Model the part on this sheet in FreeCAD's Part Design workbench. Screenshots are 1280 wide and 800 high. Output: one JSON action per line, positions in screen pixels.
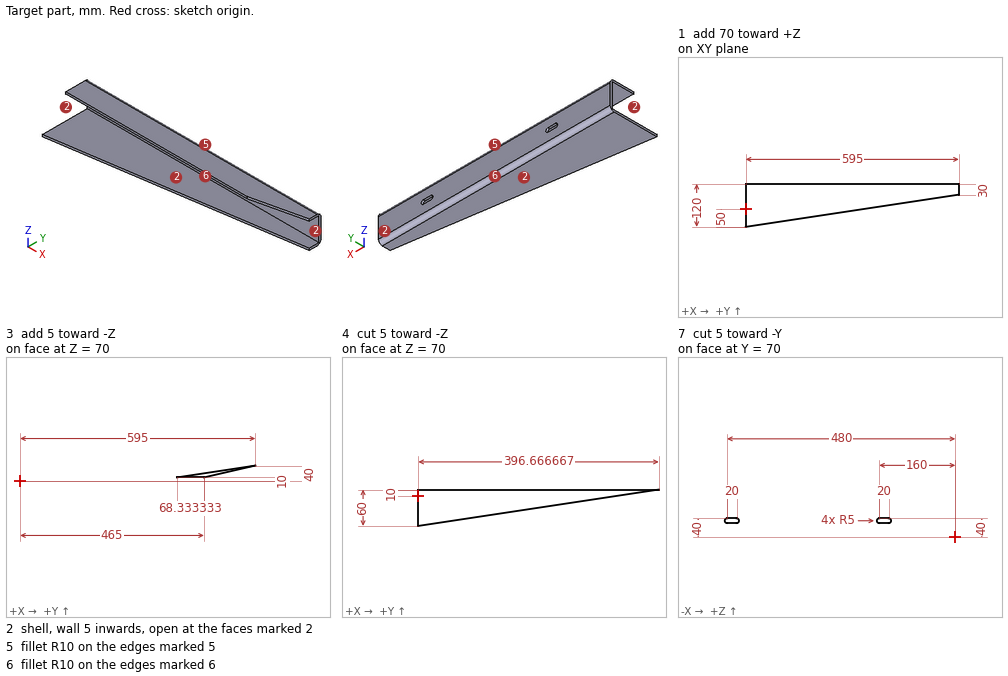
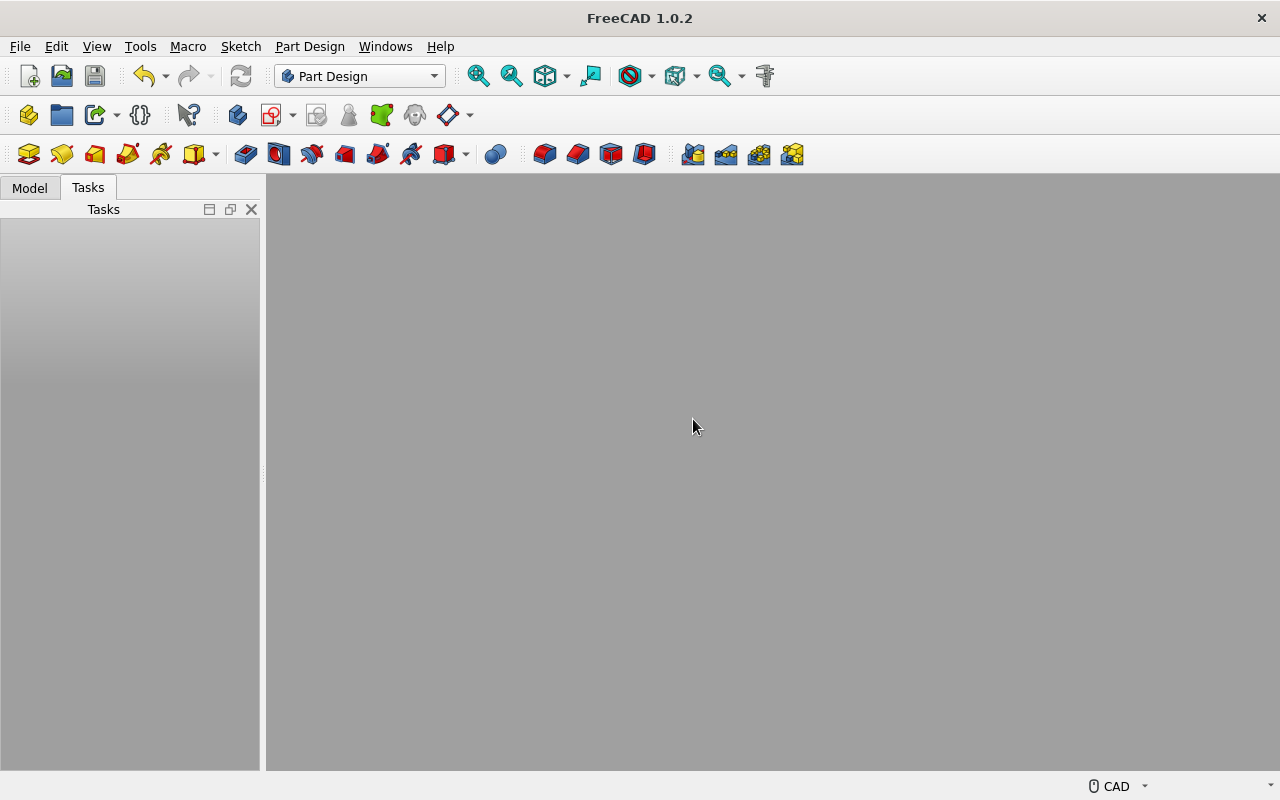
{"action": "key", "text": "ctrl+n"}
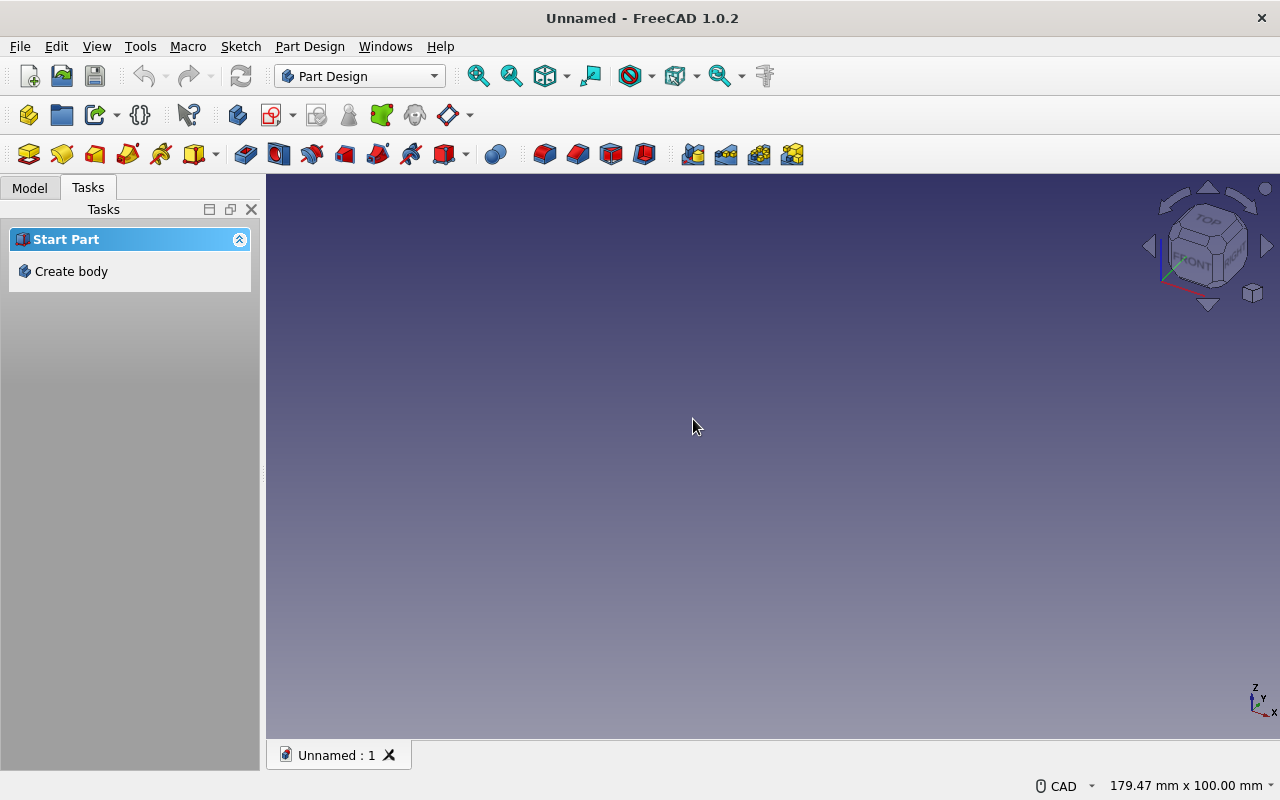
{"action": "left_click", "coordinate": [270, 116]}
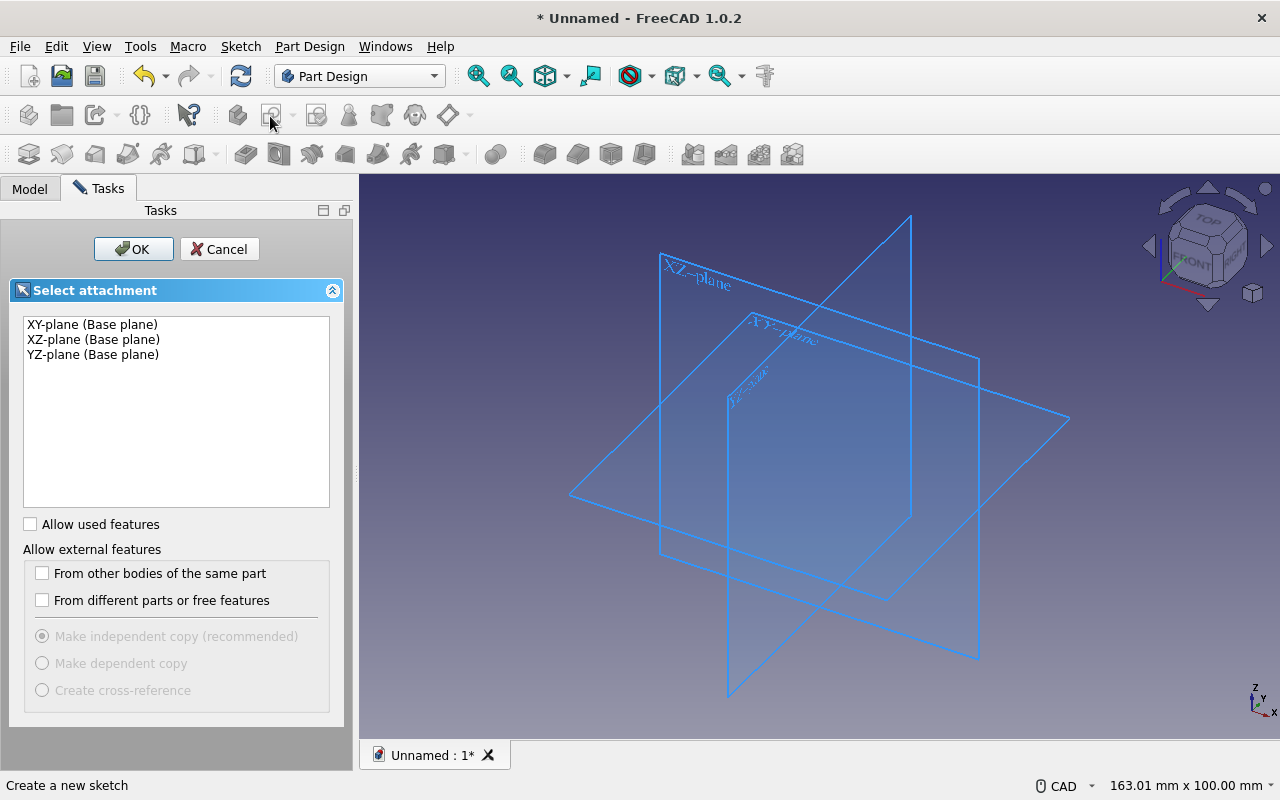
{"action": "left_click", "coordinate": [84, 324]}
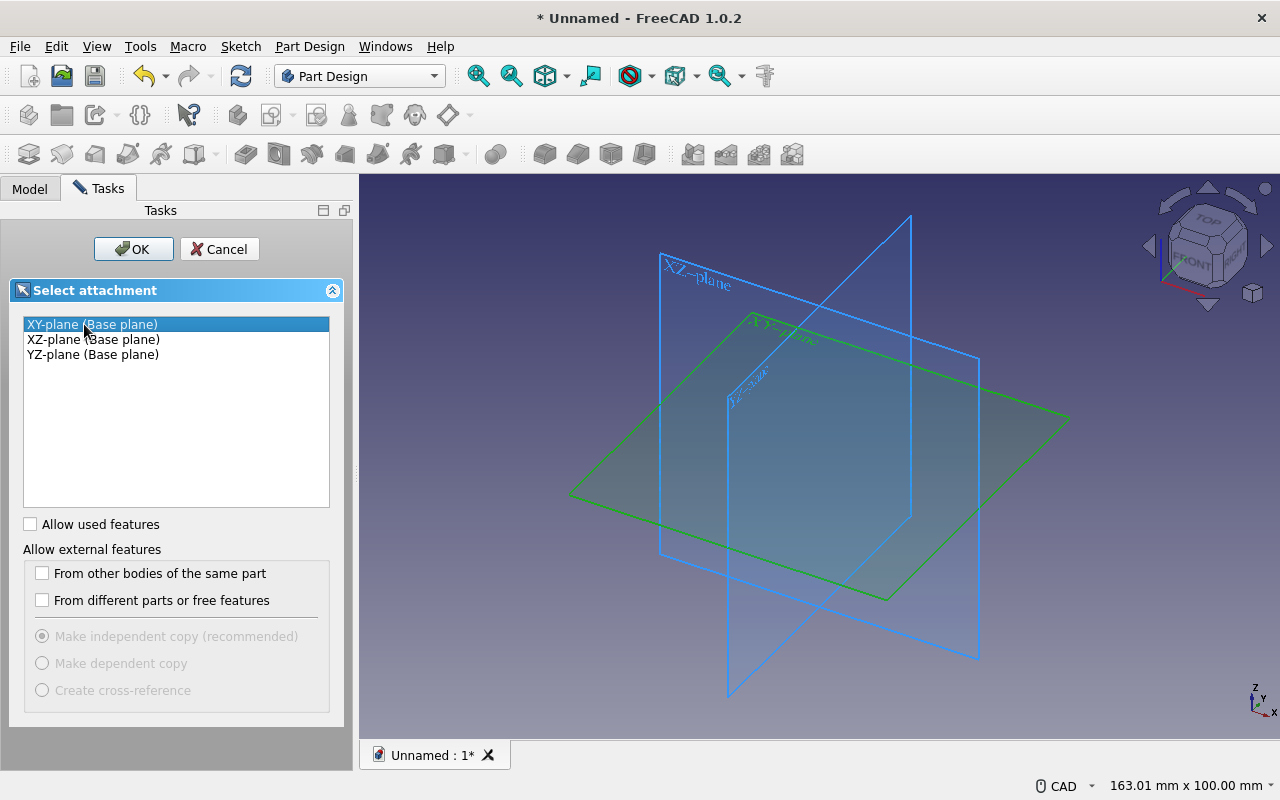
{"action": "left_click", "coordinate": [134, 249]}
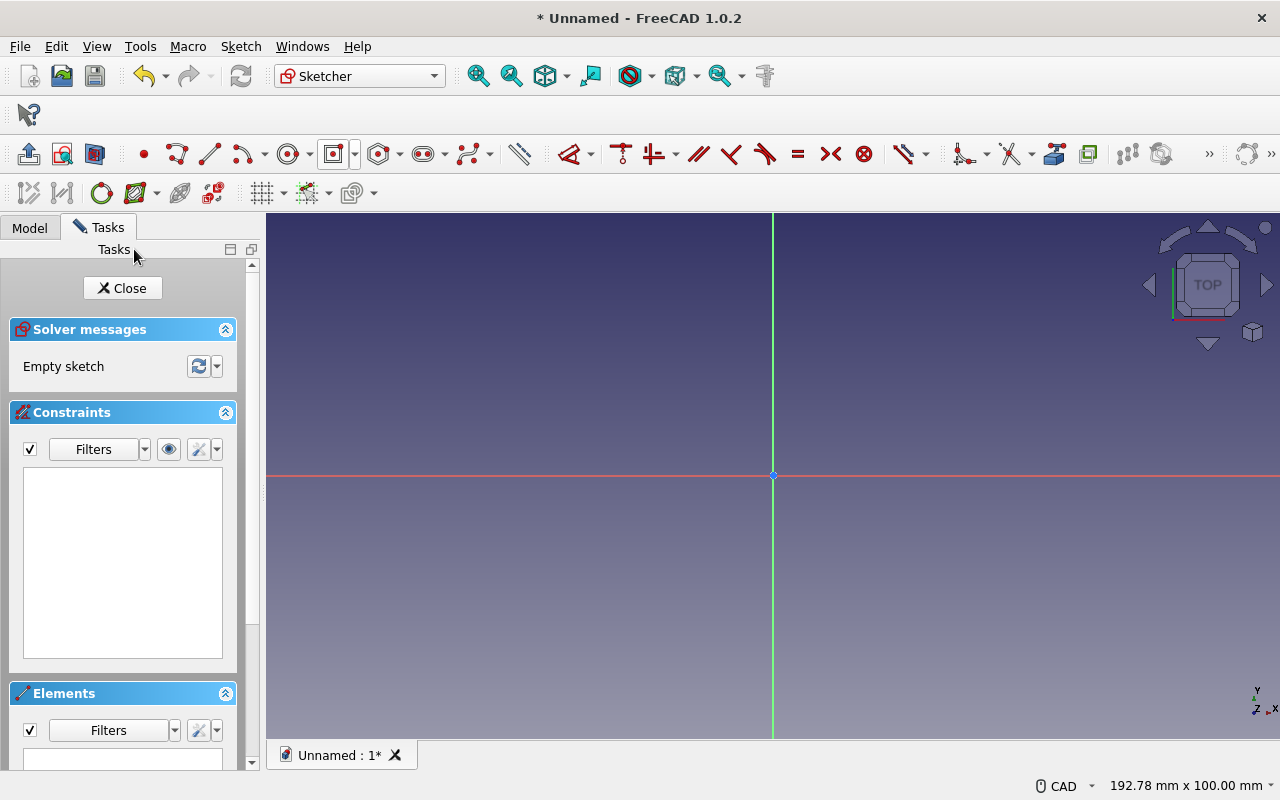
{"action": "scroll", "coordinate": [294, 489], "scroll_direction": "down", "scroll_amount": 8}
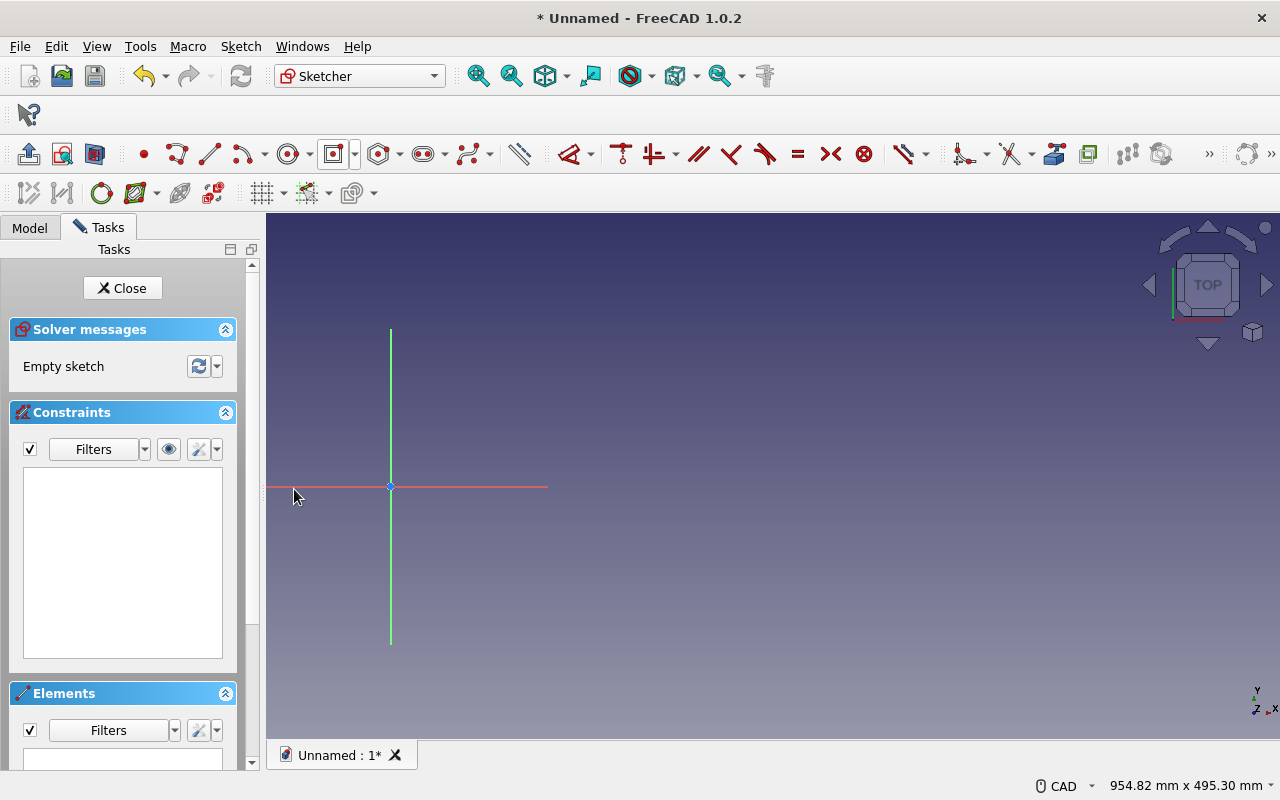
{"action": "key", "text": "g m"}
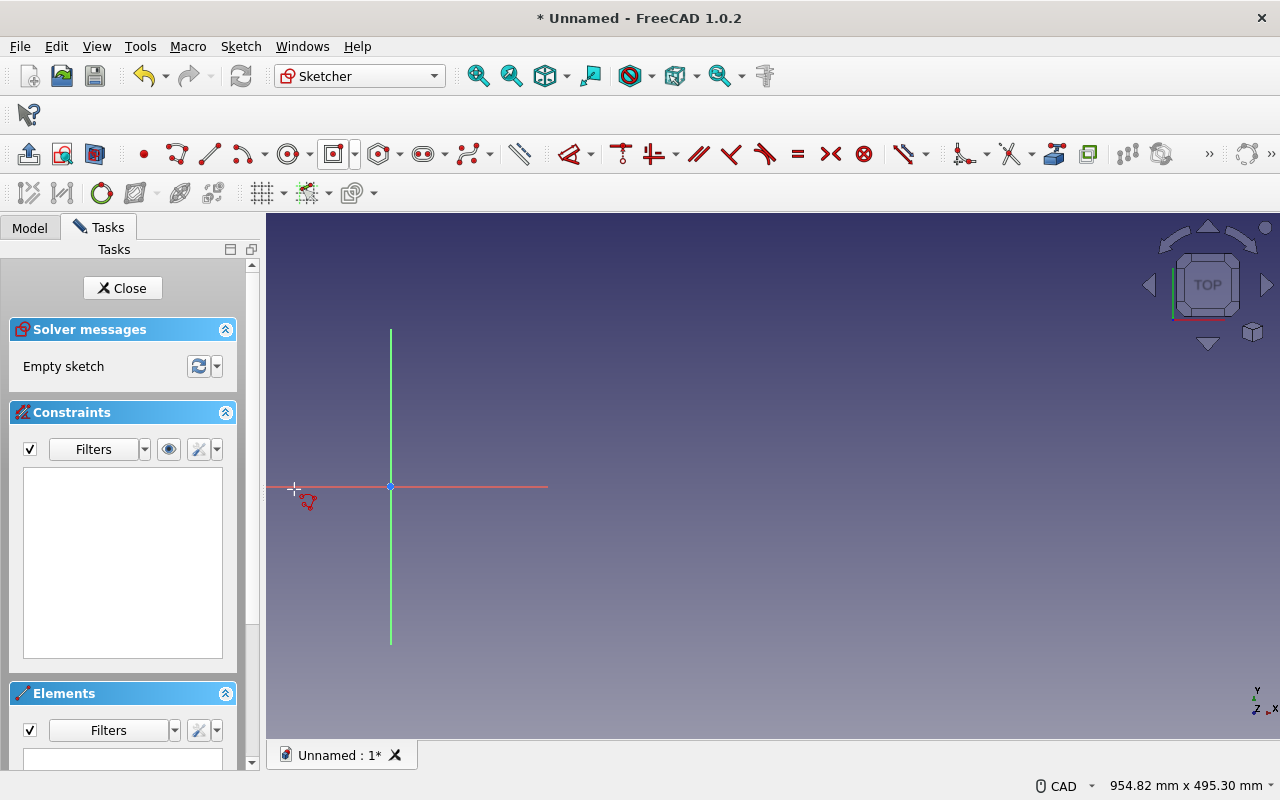
{"action": "left_click", "coordinate": [391, 540]}
{"action": "left_click", "coordinate": [1023, 444]}
{"action": "left_click", "coordinate": [1023, 412]}
{"action": "left_click", "coordinate": [400, 412]}
{"action": "left_click", "coordinate": [391, 541]}
{"action": "key", "text": "Escape"}
{"action": "key", "text": "Escape"}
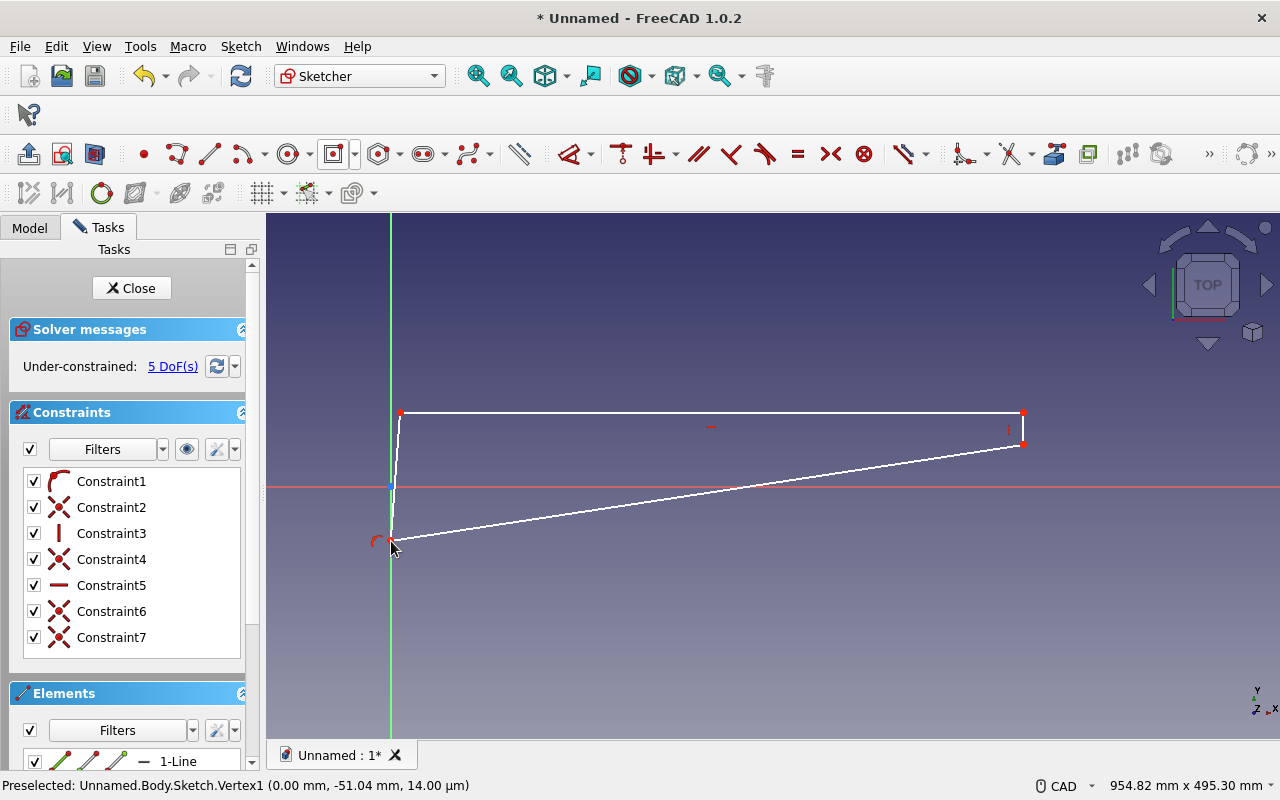
{"action": "left_click", "coordinate": [394, 503]}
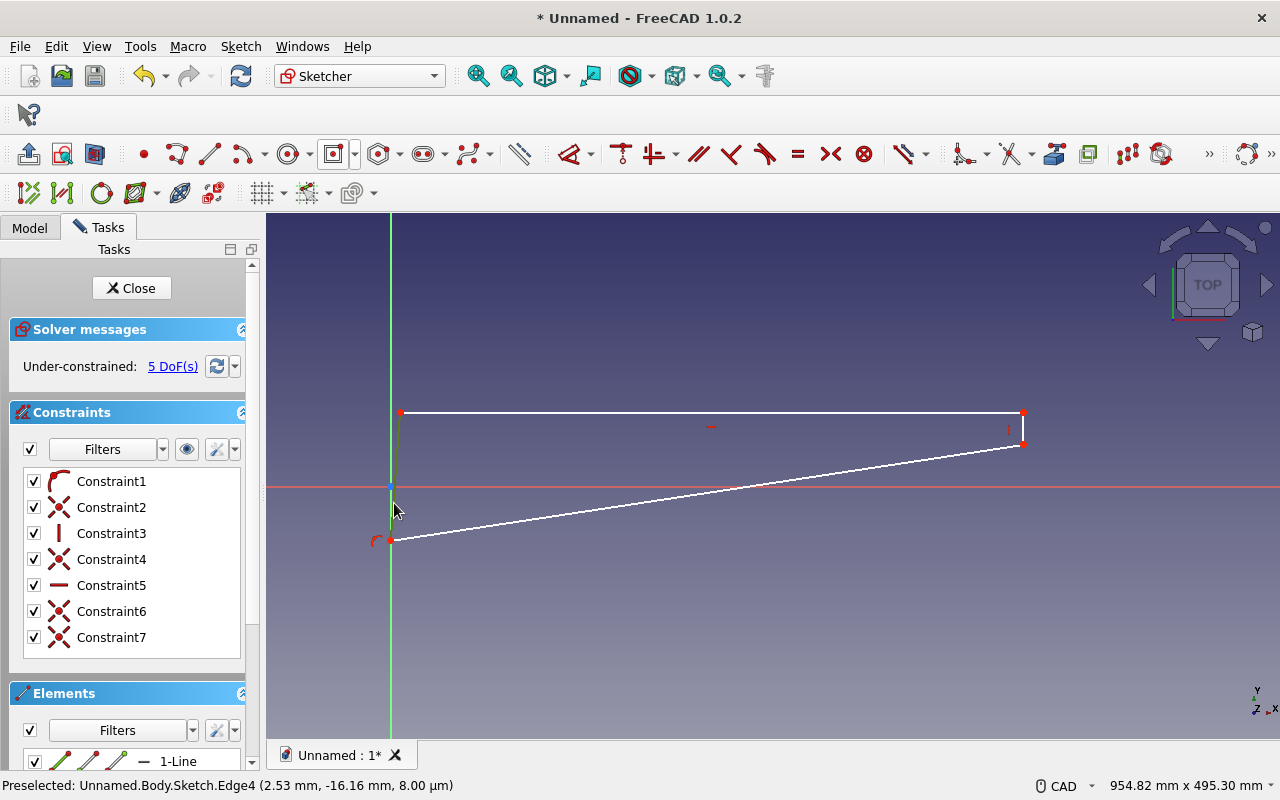
{"action": "key", "text": "v"}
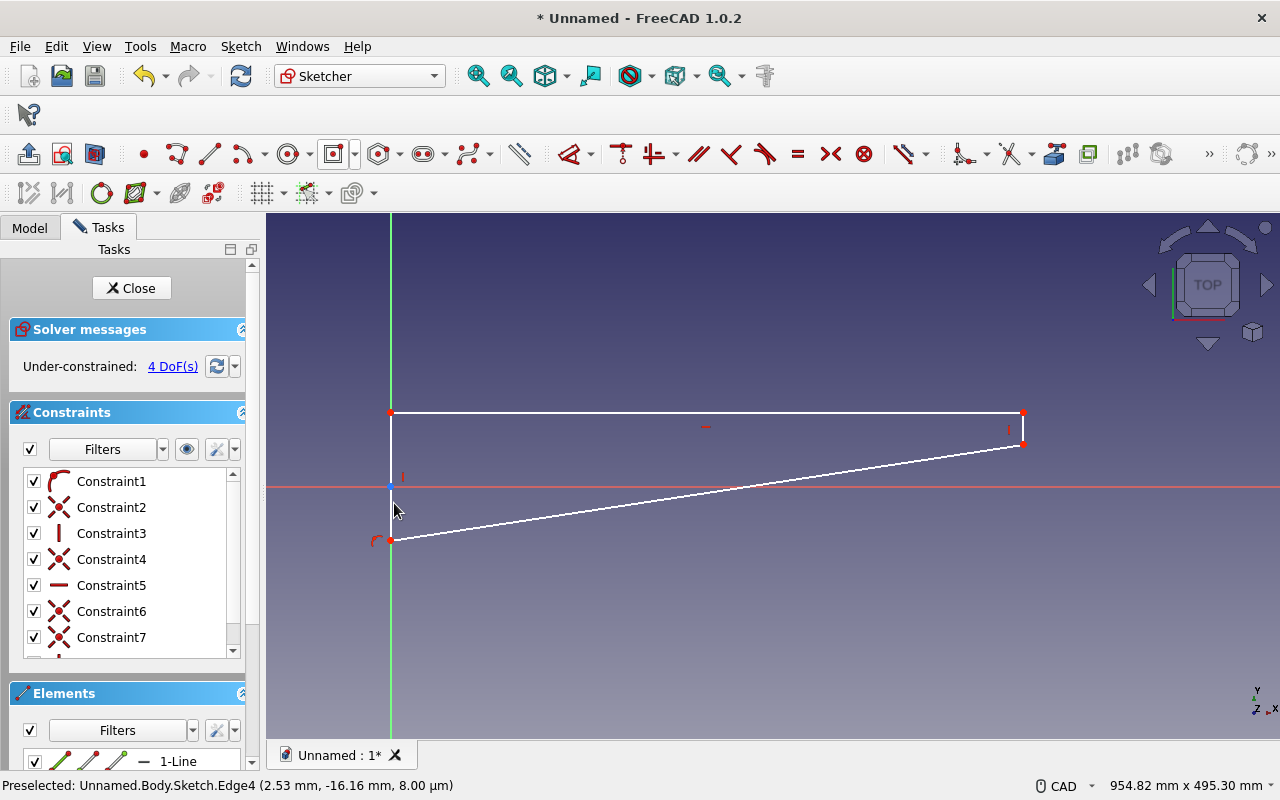
{"action": "scroll", "coordinate": [1023, 435], "scroll_direction": "up", "scroll_amount": 2}